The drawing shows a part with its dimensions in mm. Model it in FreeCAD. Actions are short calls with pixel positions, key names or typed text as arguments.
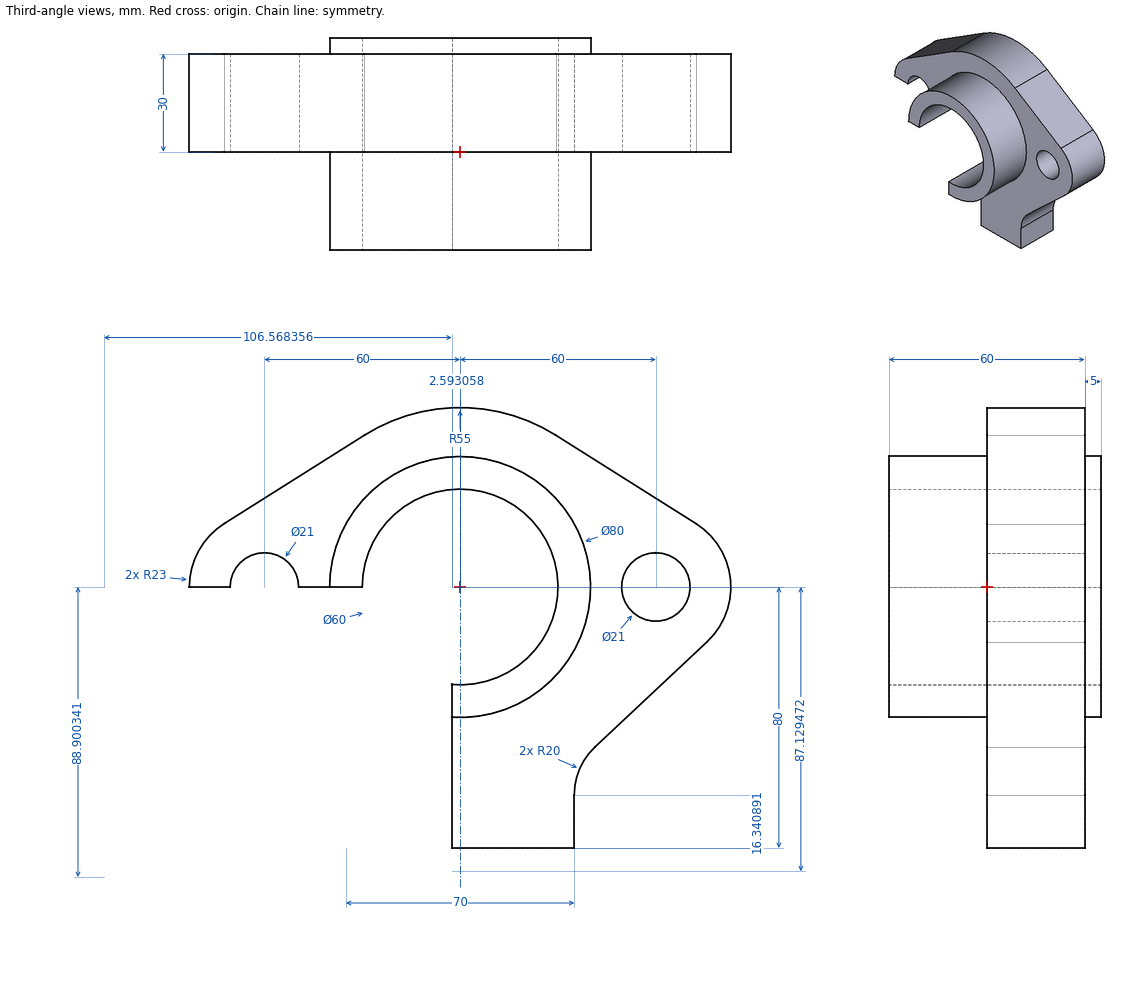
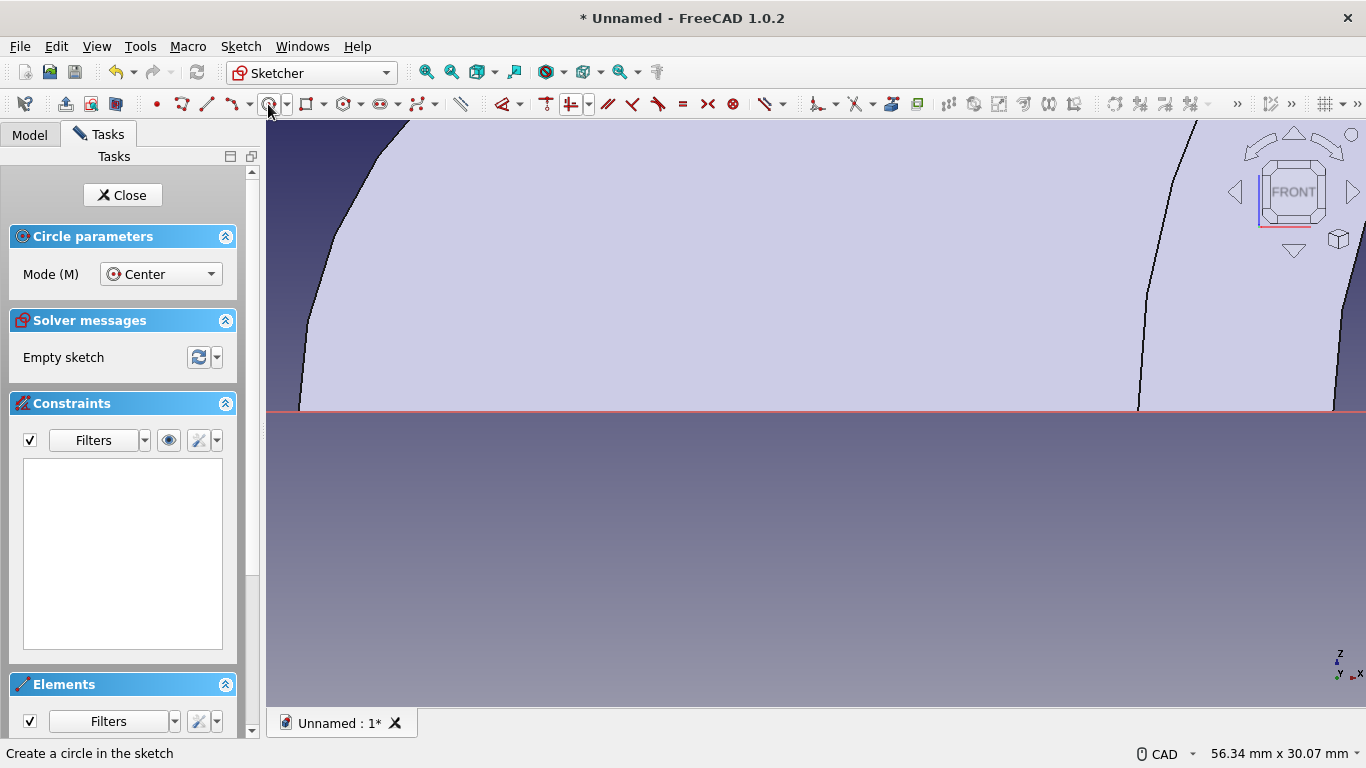
click(748, 412)
move(893, 267)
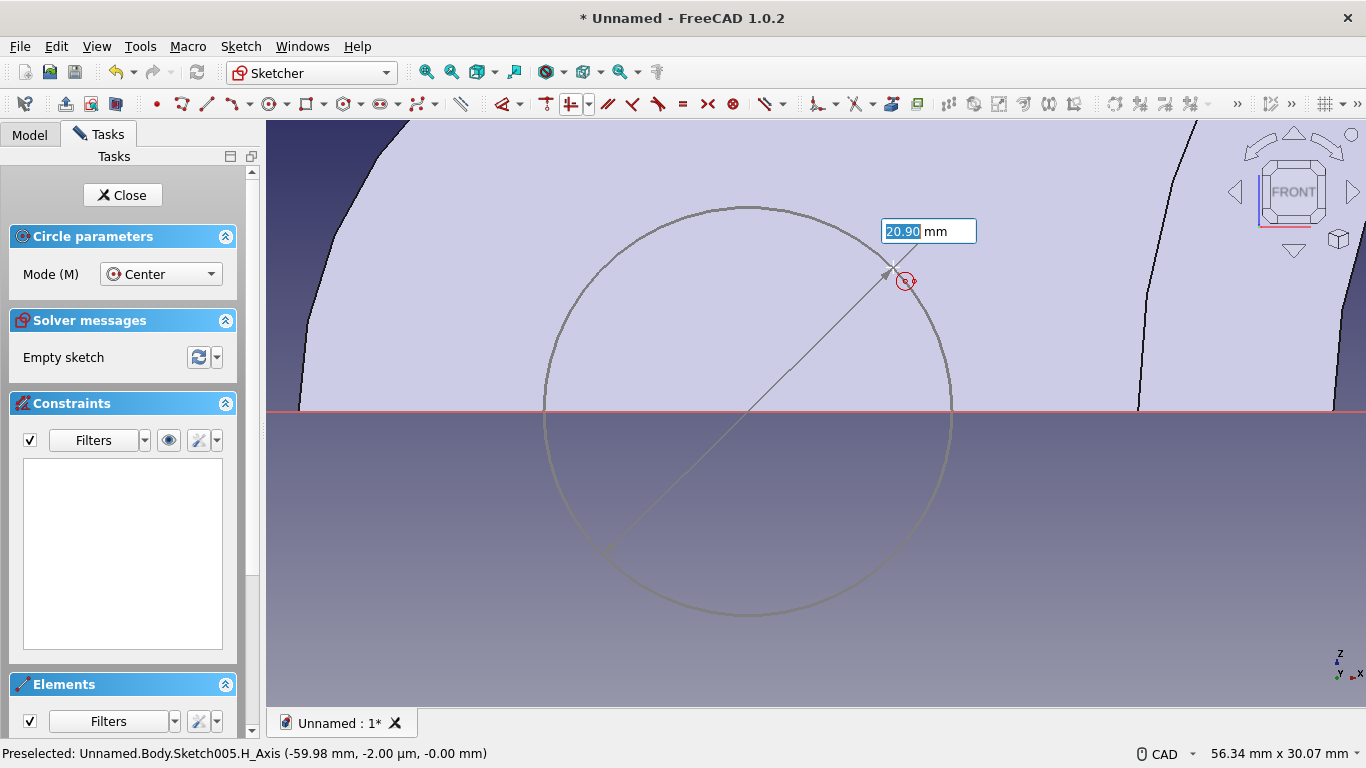
text(21)
key(Return)
key(Escape)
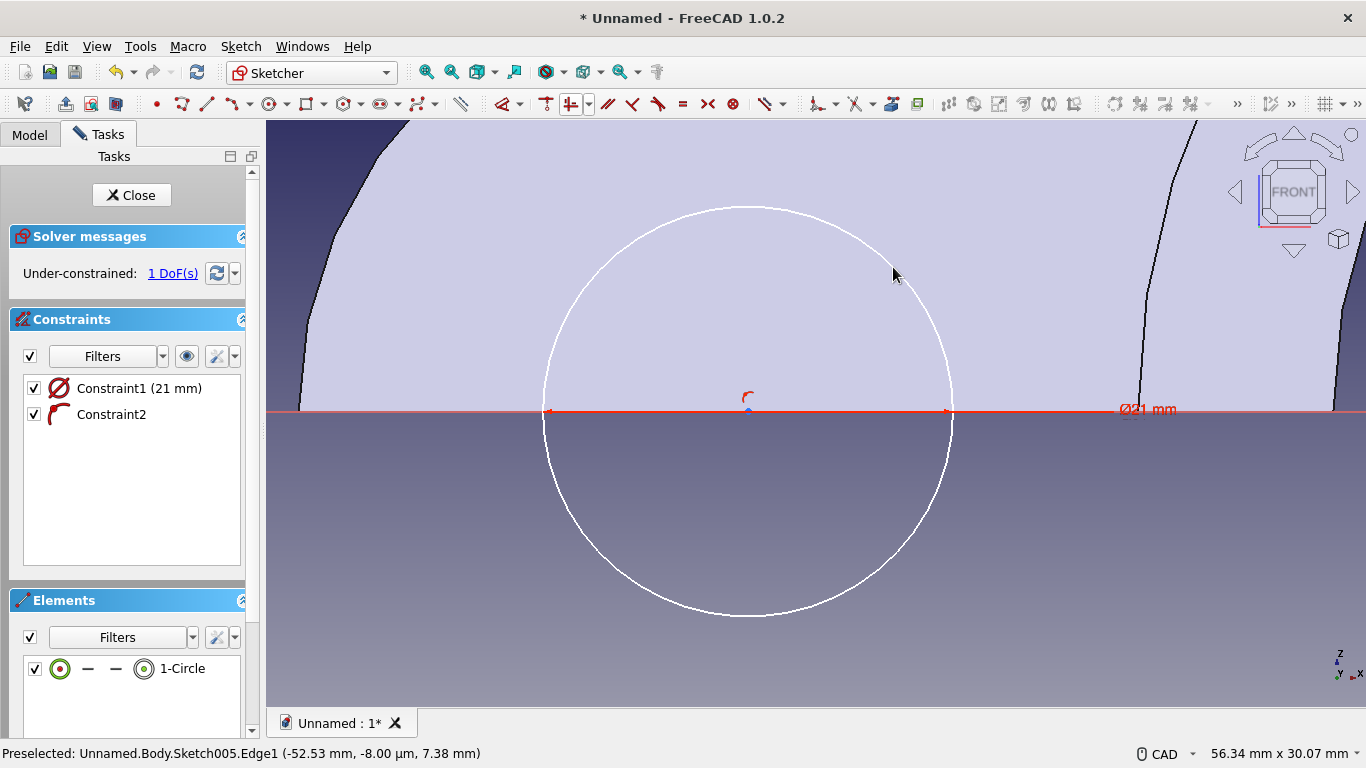
click(502, 104)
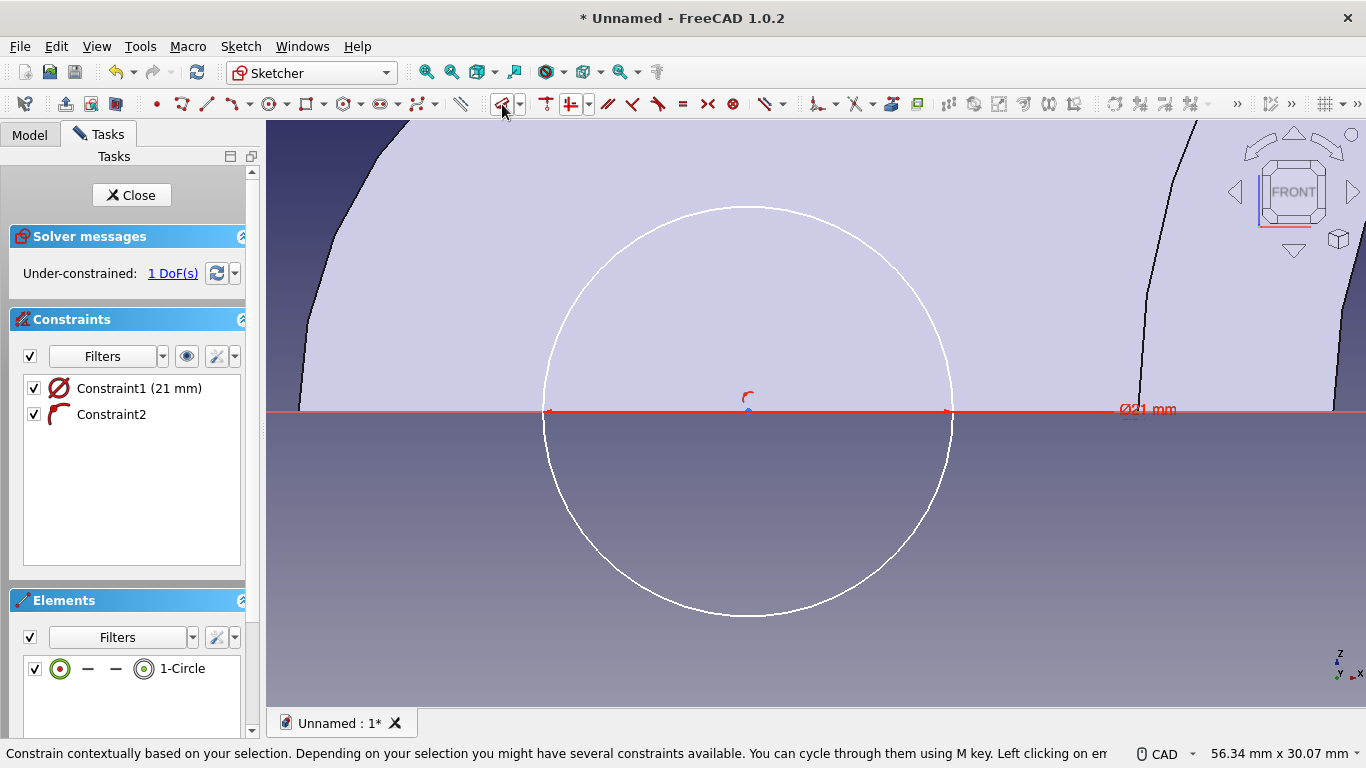
click(748, 412)
click(975, 446)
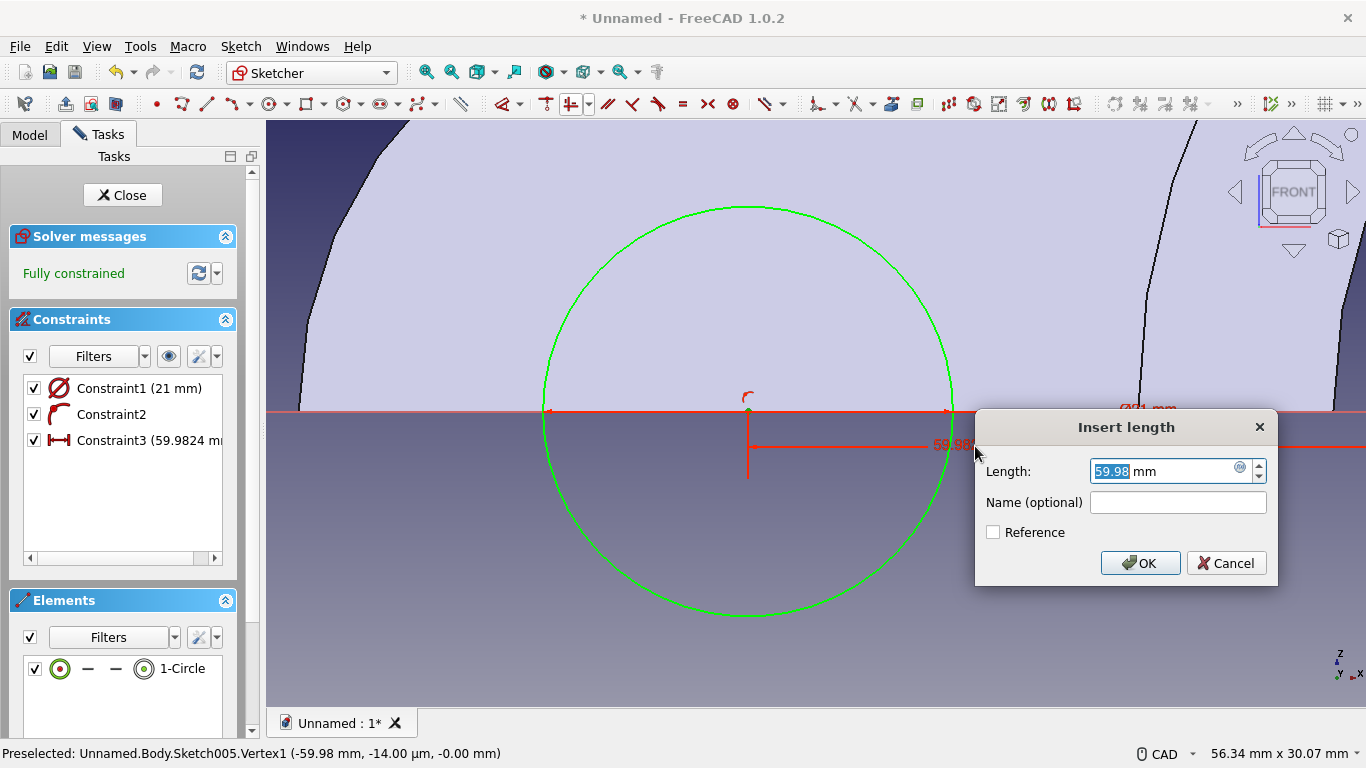
text(60)
key(Return)
key(Escape)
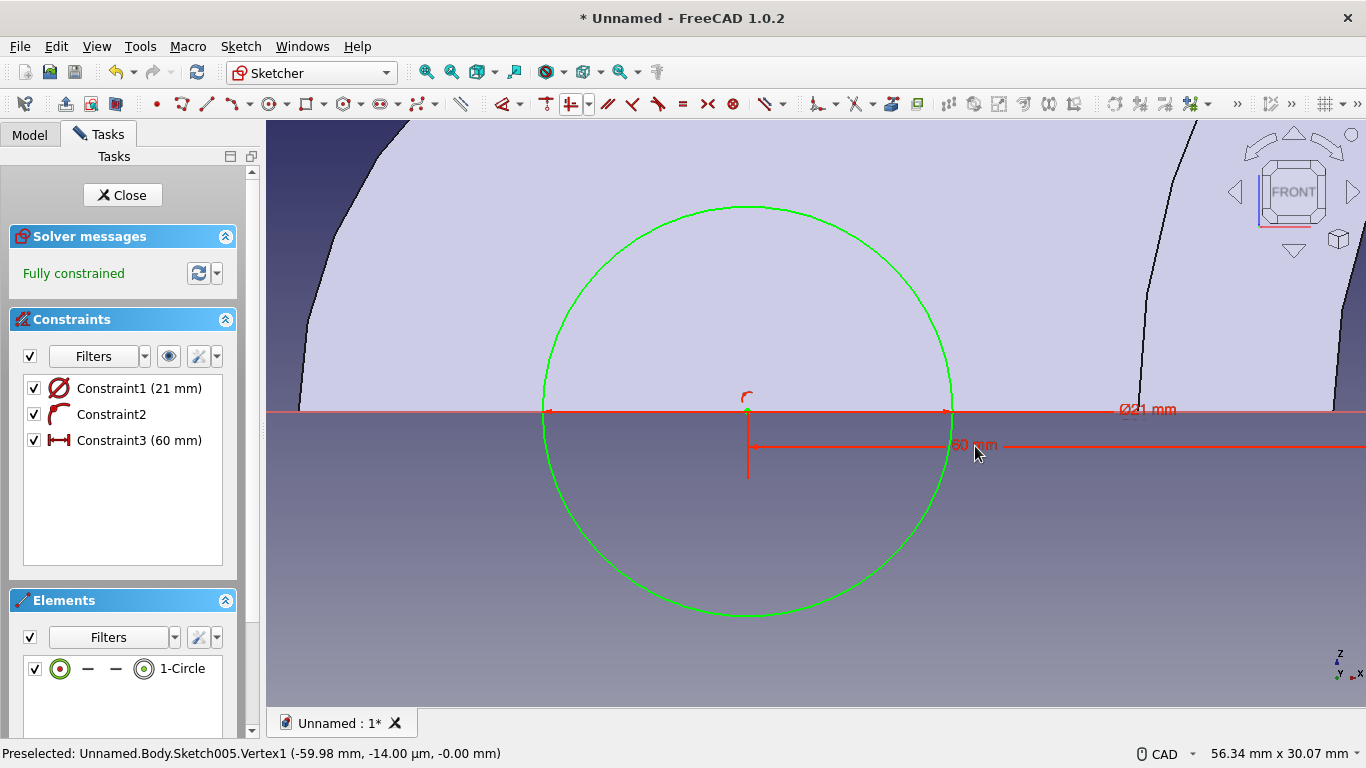
click(123, 195)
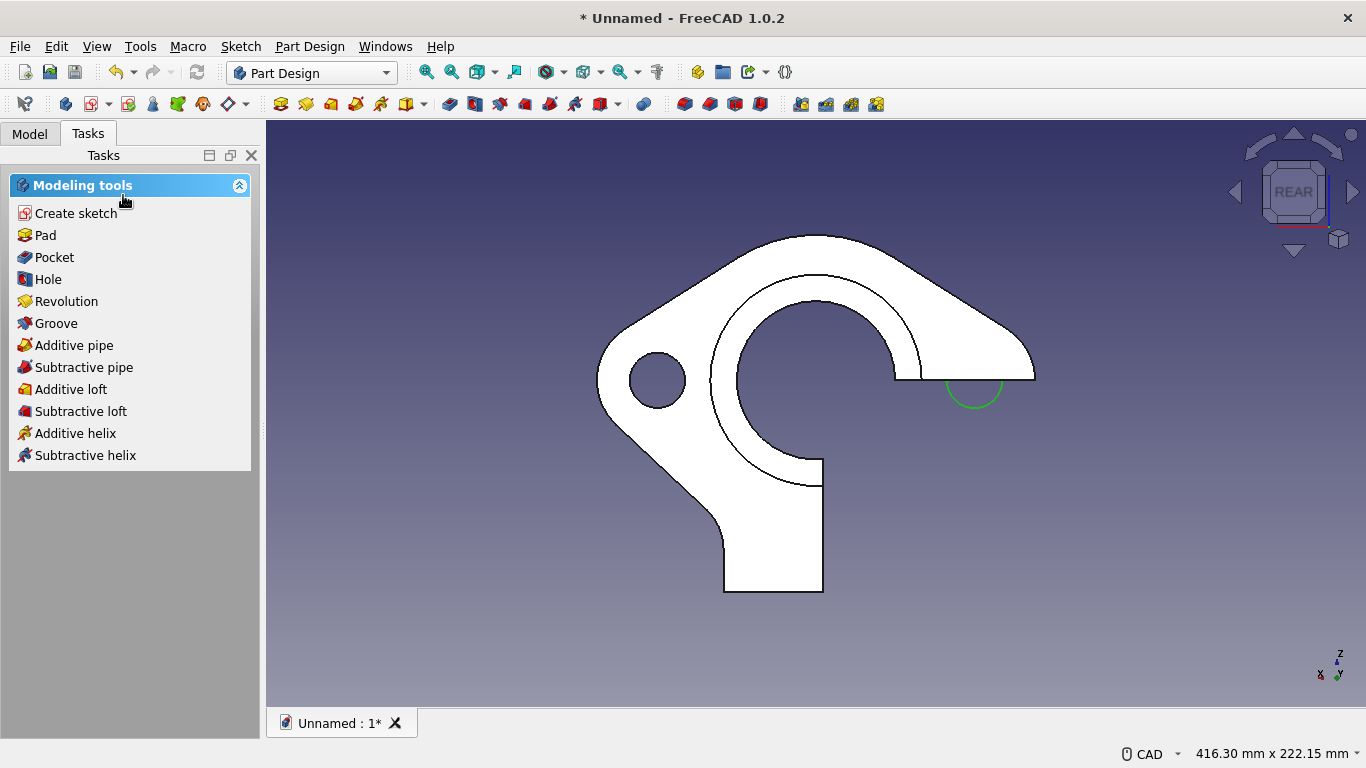
click(450, 104)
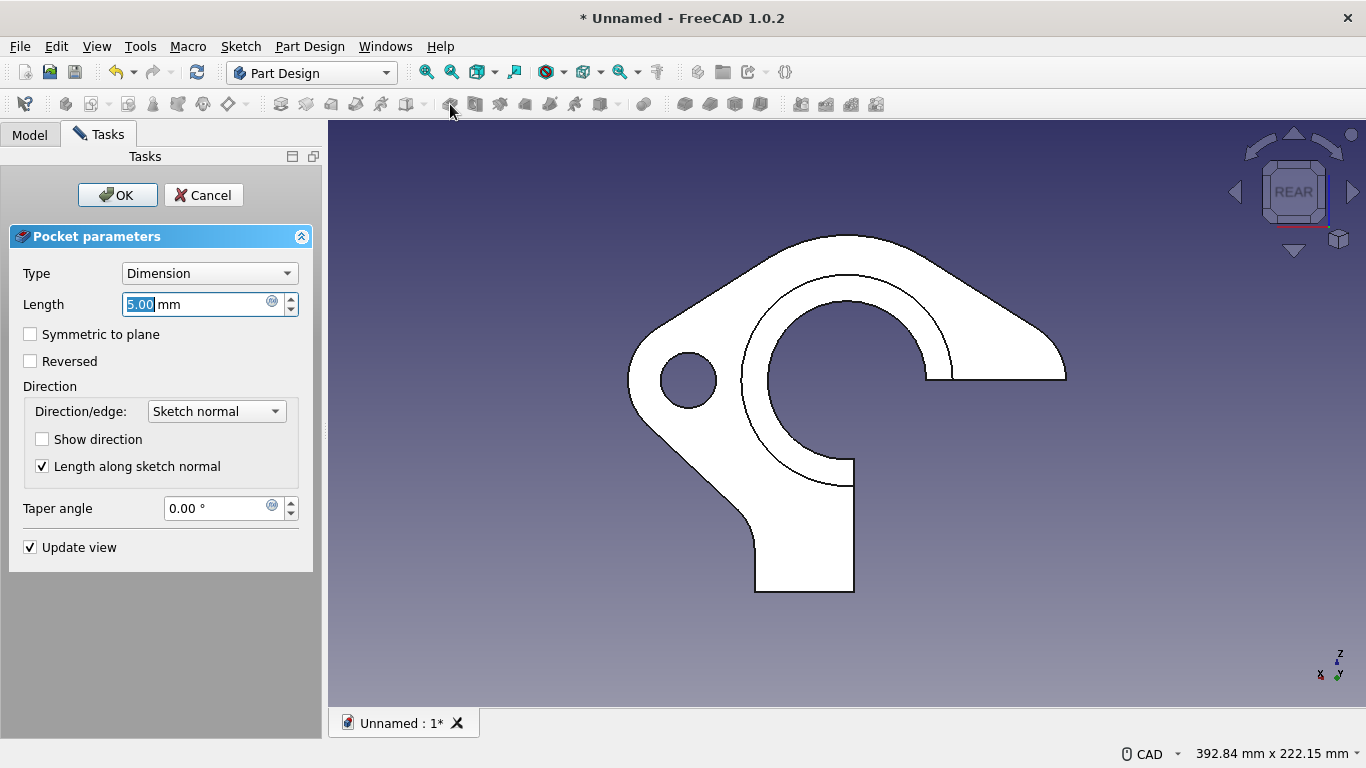
click(210, 274)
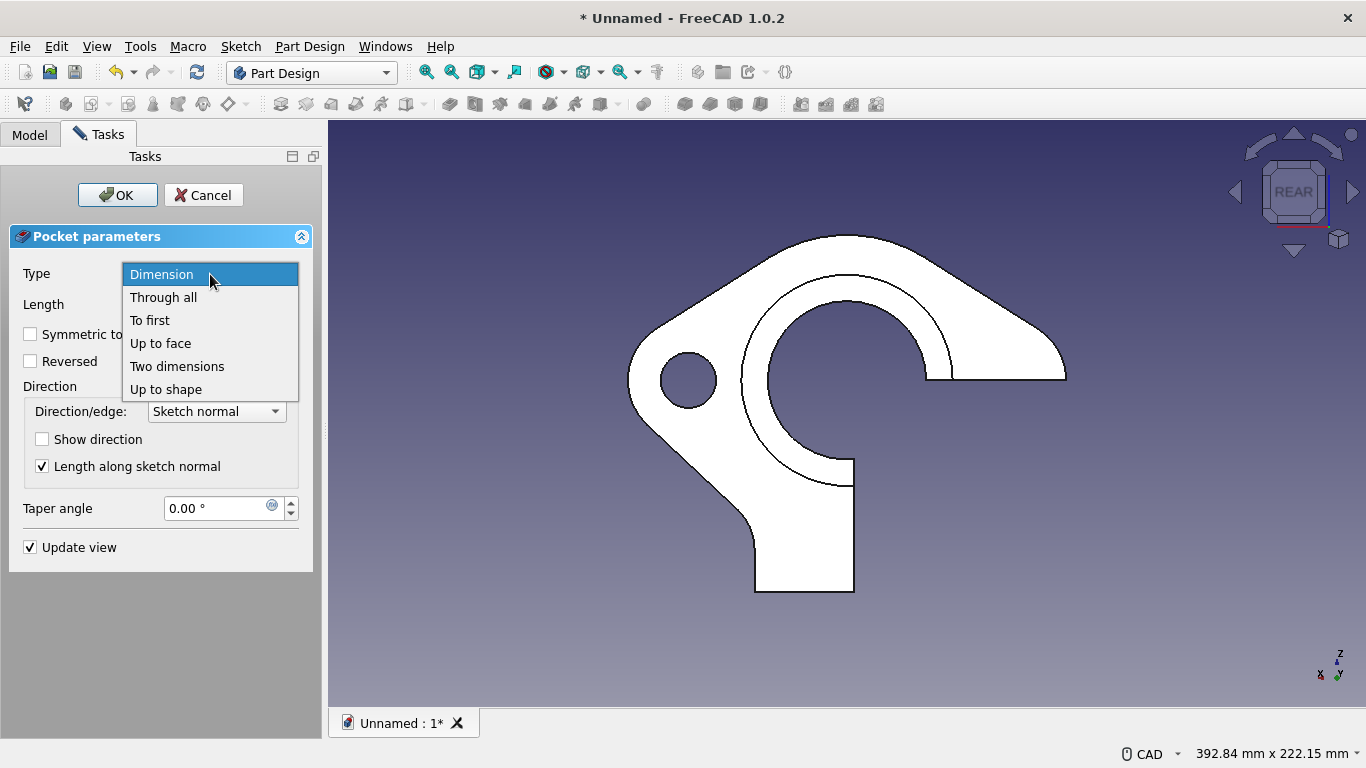
click(208, 366)